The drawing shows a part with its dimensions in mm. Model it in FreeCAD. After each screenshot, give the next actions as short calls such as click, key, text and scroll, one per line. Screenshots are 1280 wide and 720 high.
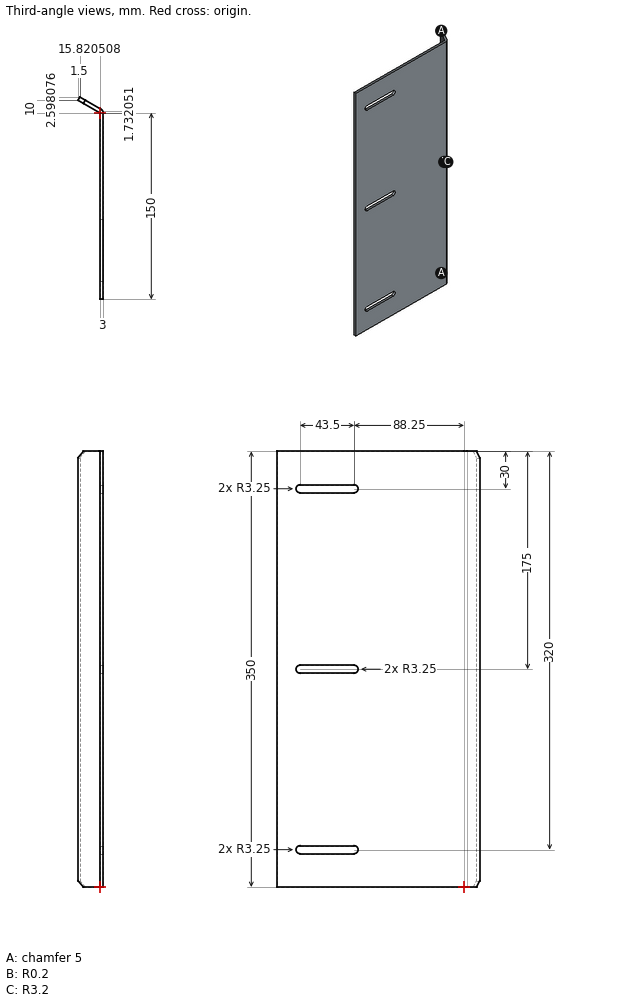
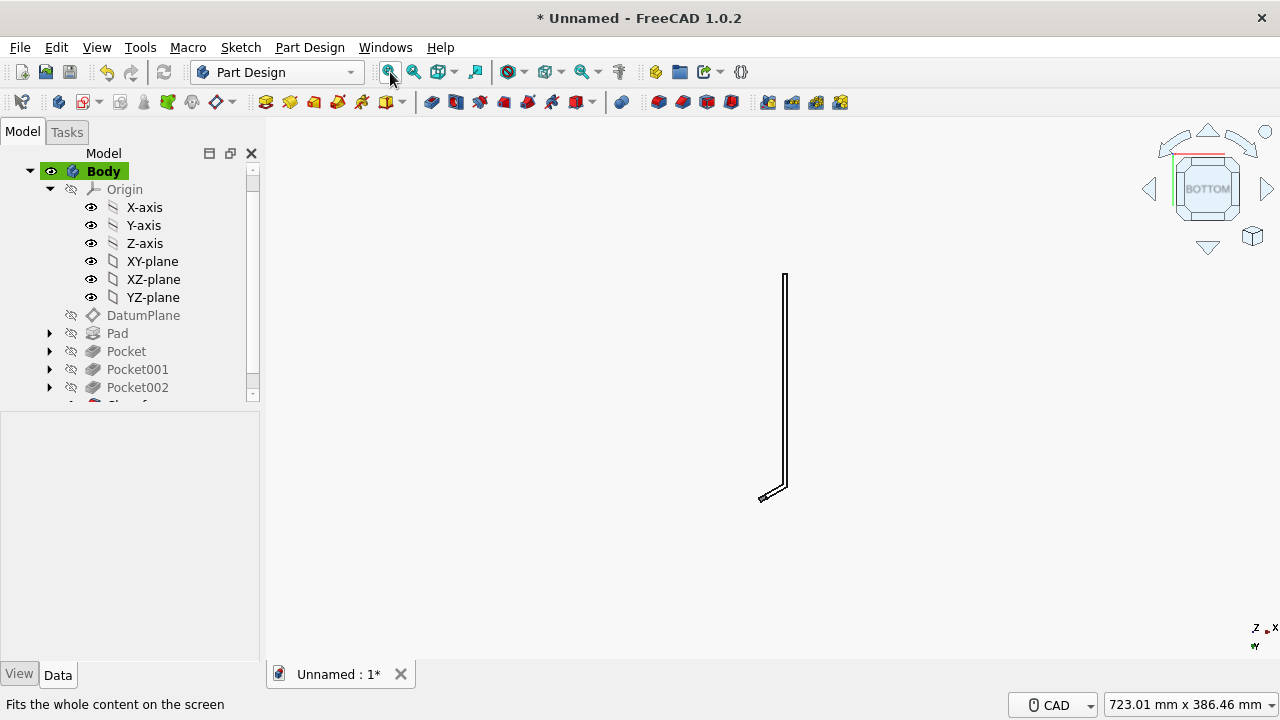
click(390, 72)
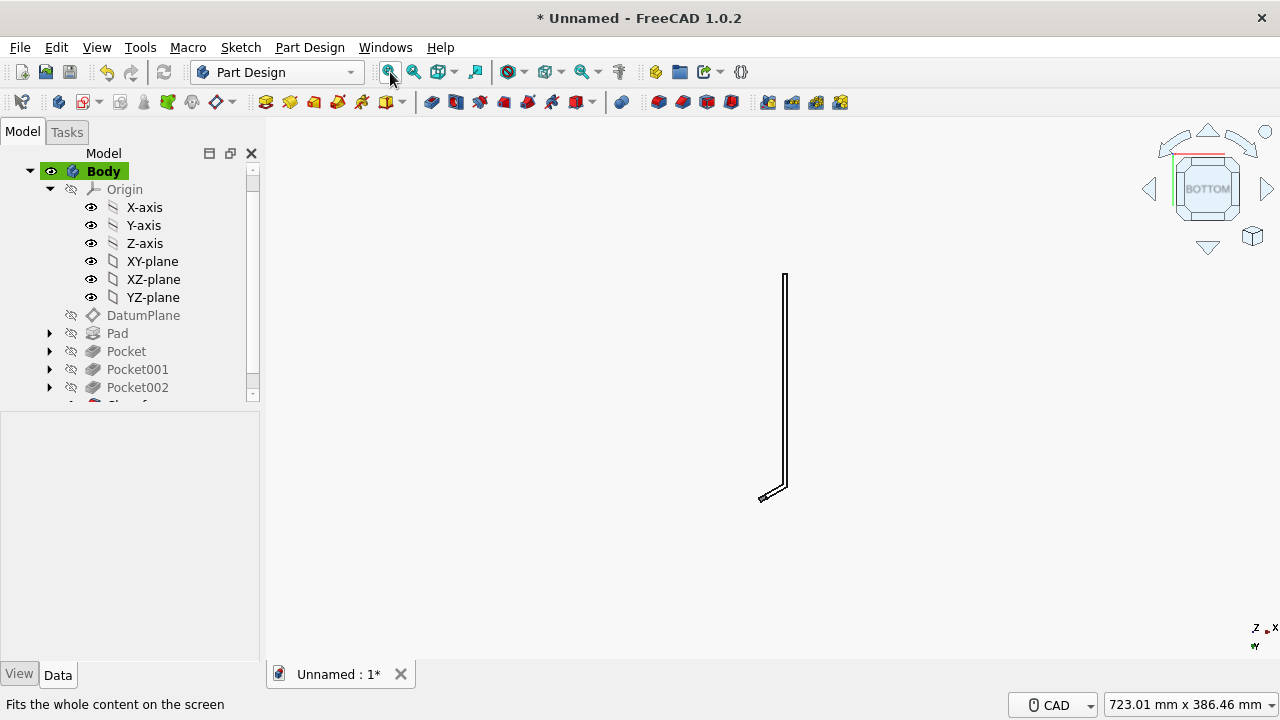
key(4)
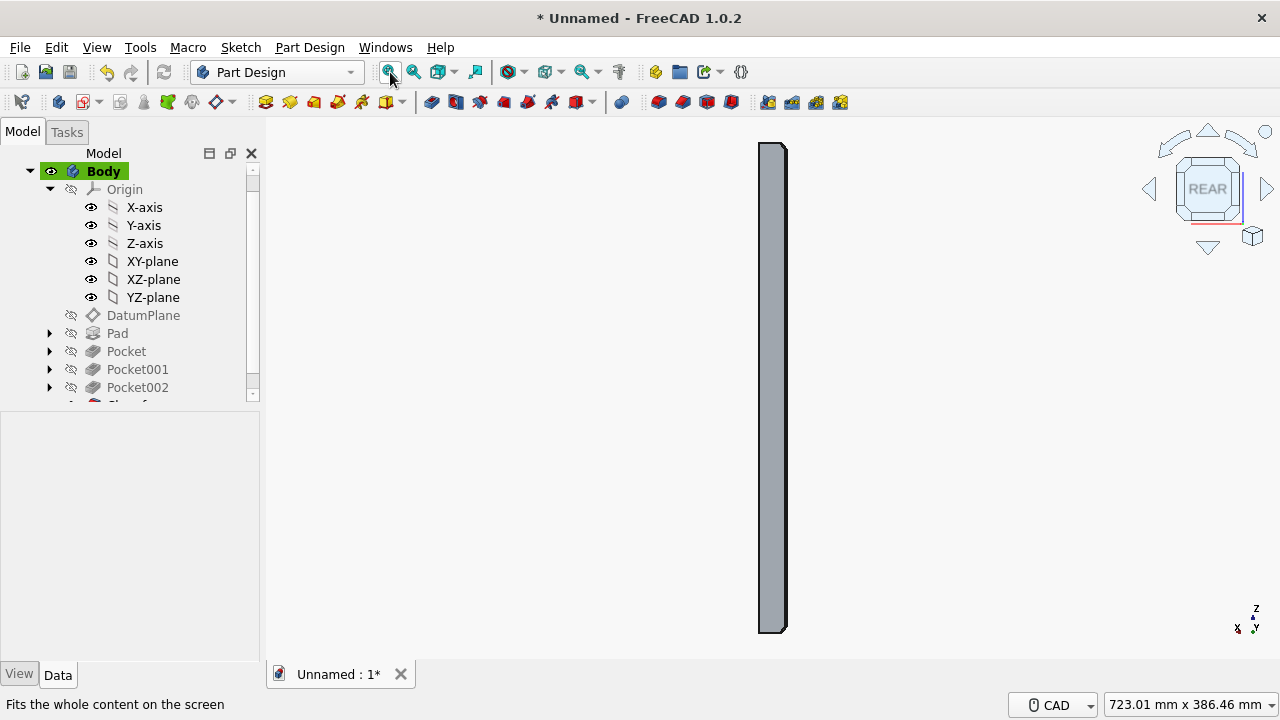
key(6)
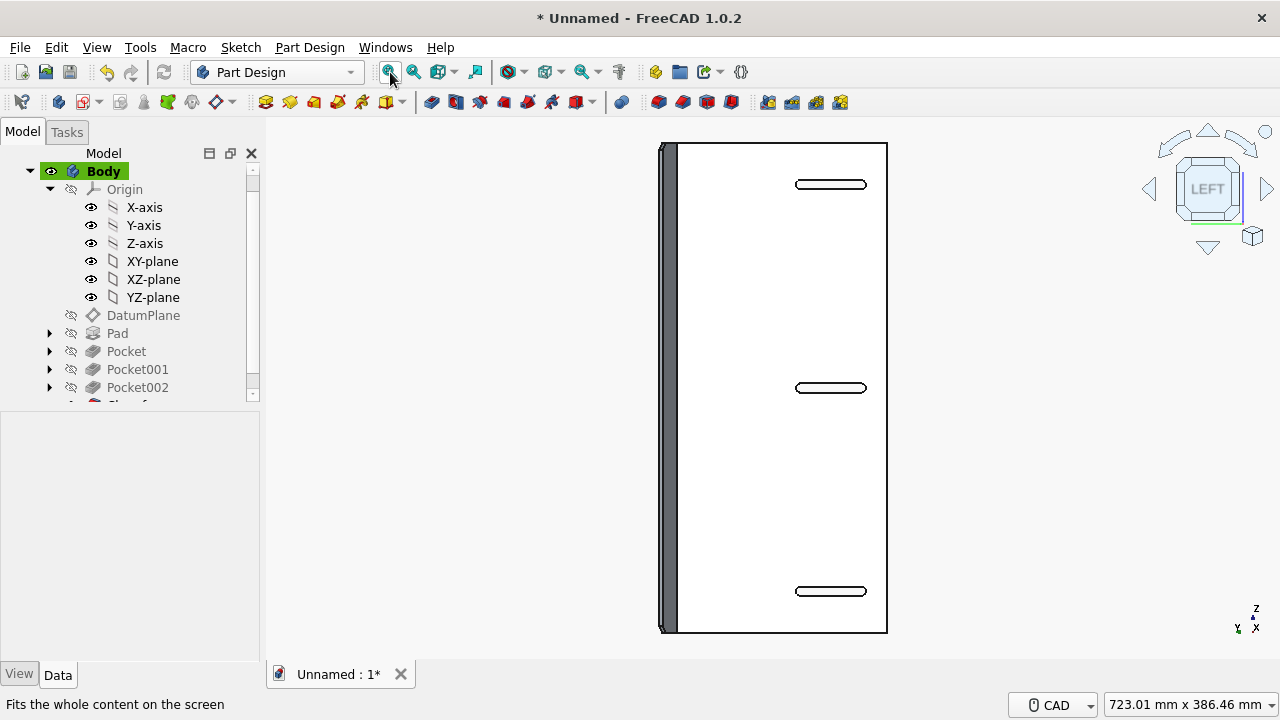
key(v)
key(3)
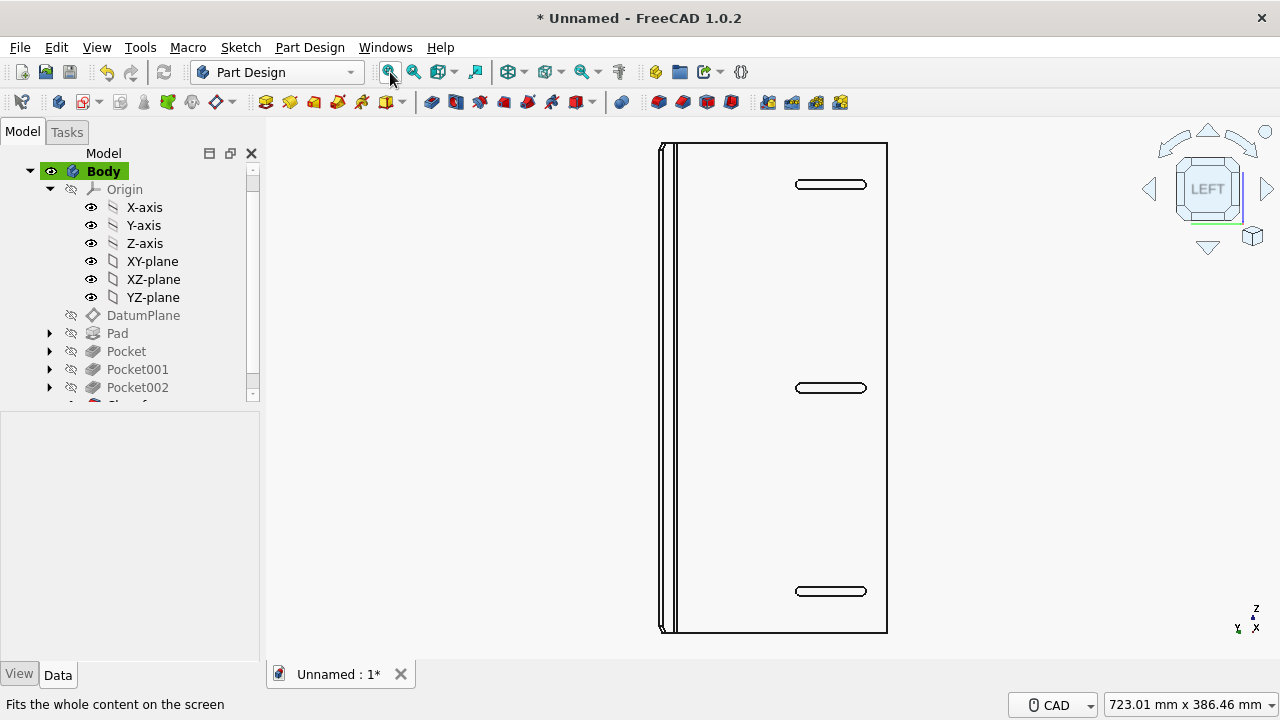
key(0)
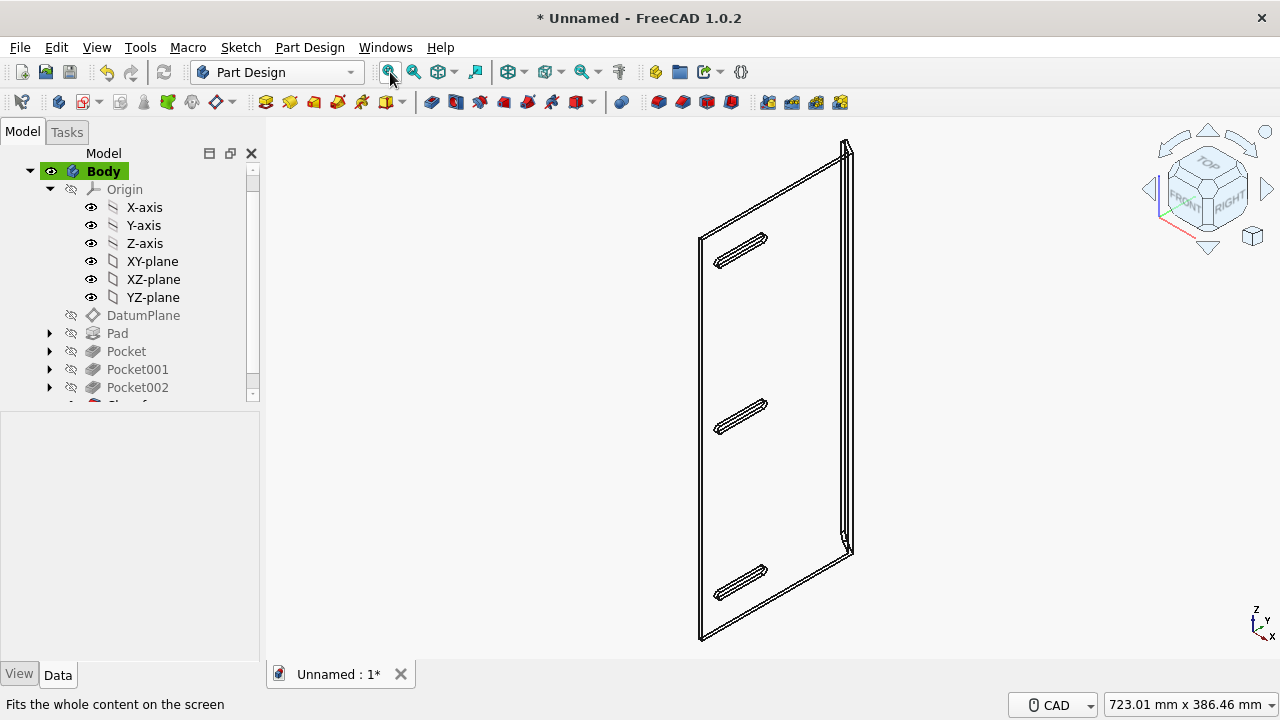
scroll(848, 352, up, 6)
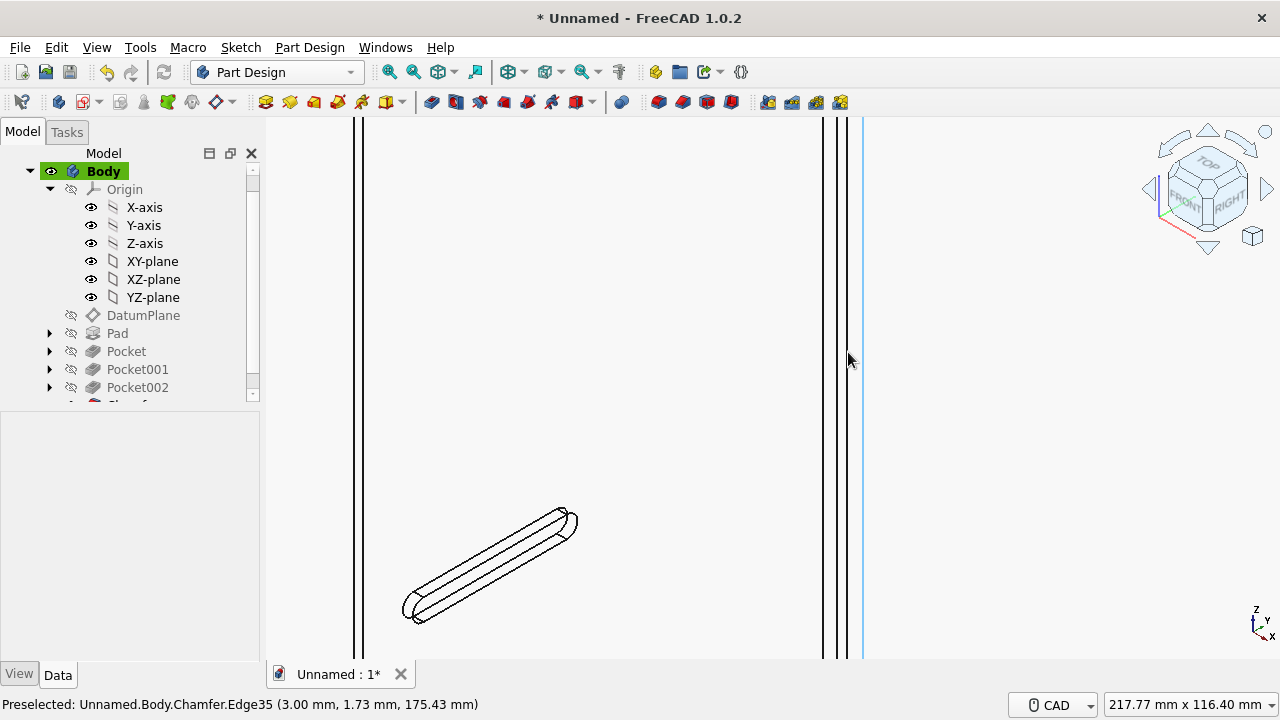
click(847, 353)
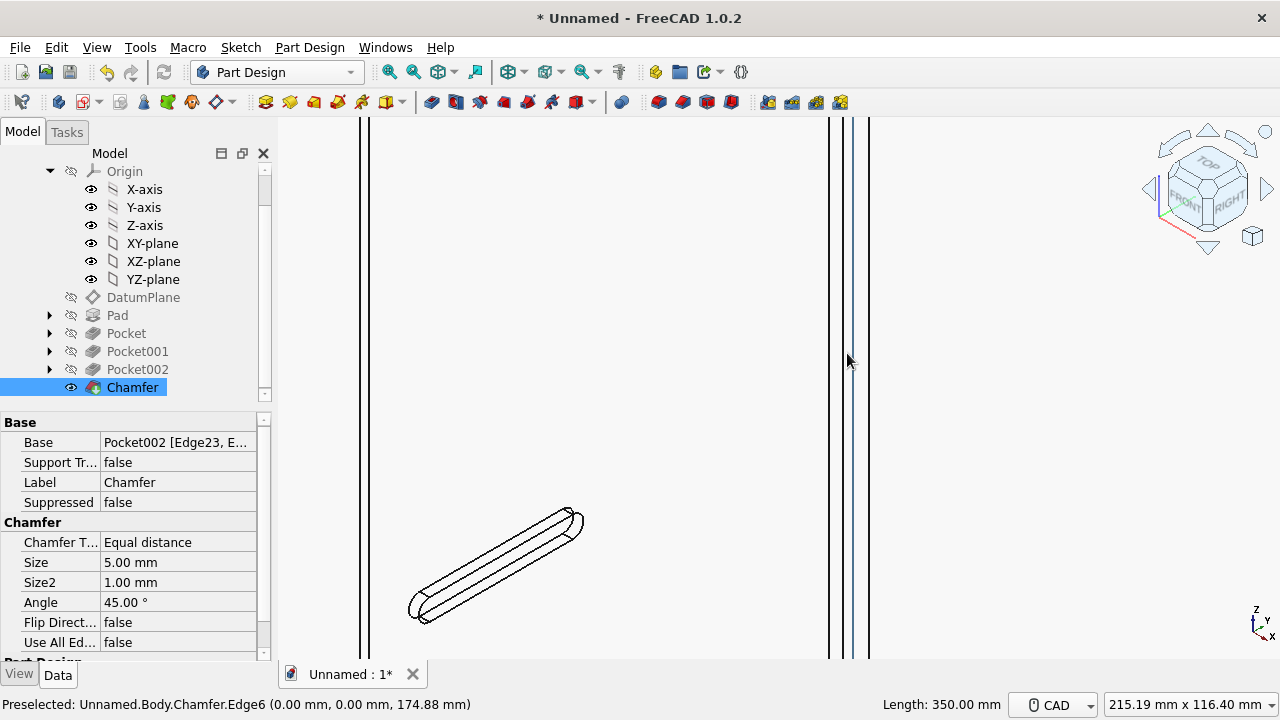
key(v)
key(1)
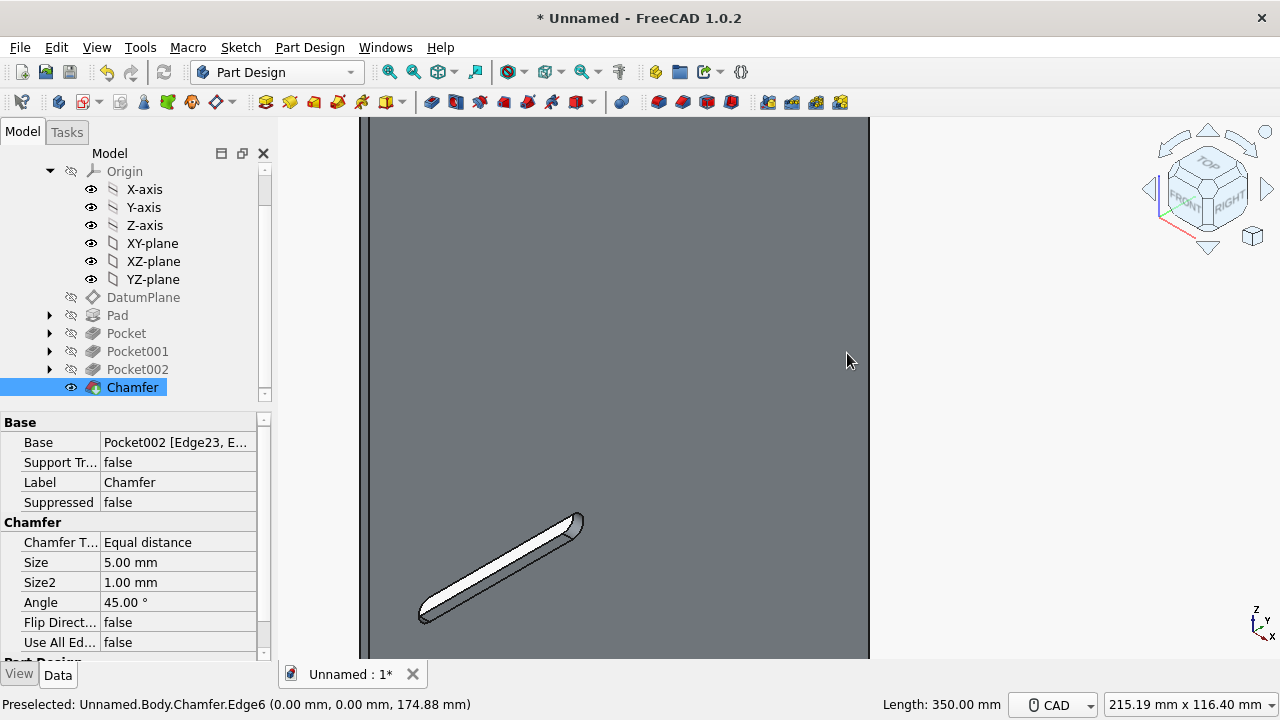
click(660, 102)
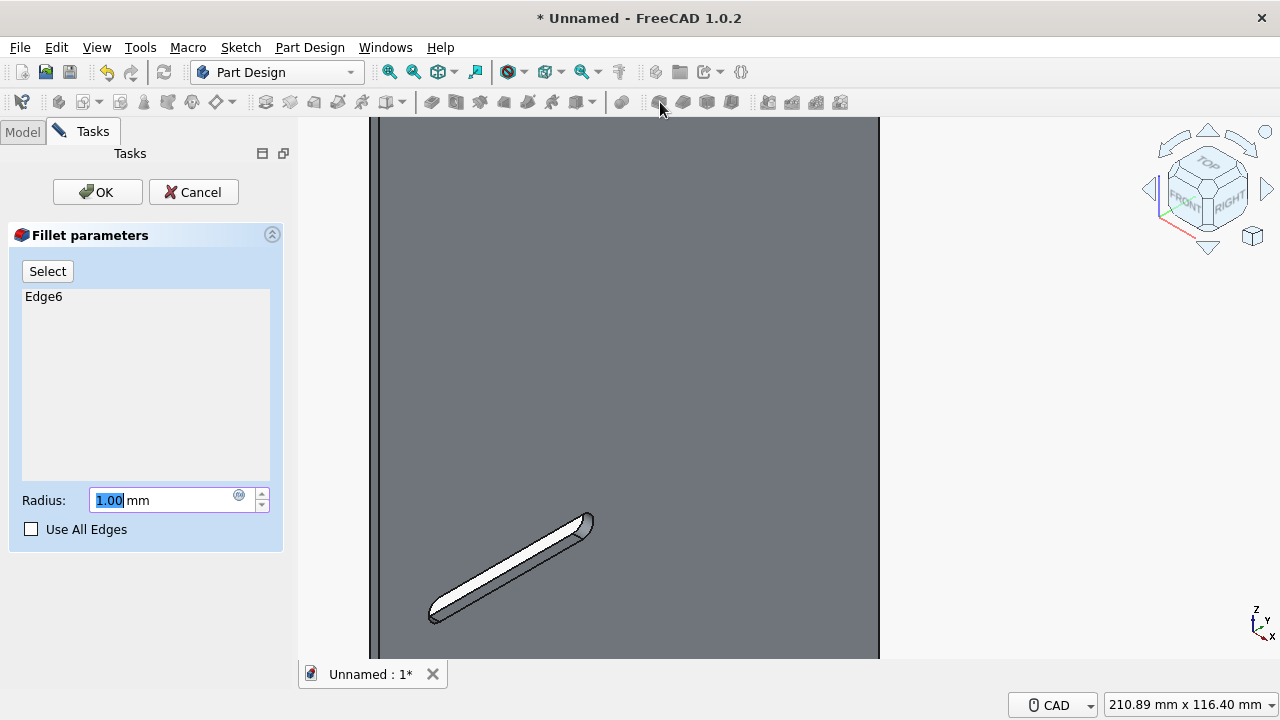
text(0.2)
key(Tab)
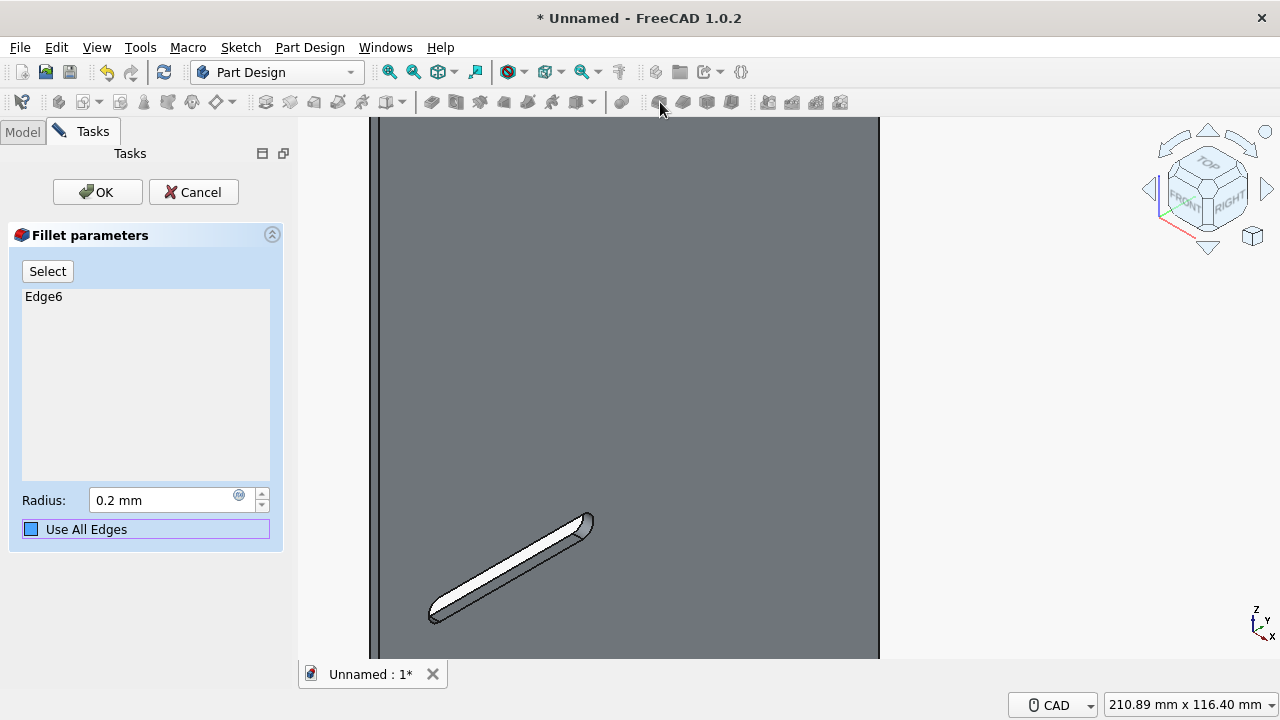
click(98, 192)